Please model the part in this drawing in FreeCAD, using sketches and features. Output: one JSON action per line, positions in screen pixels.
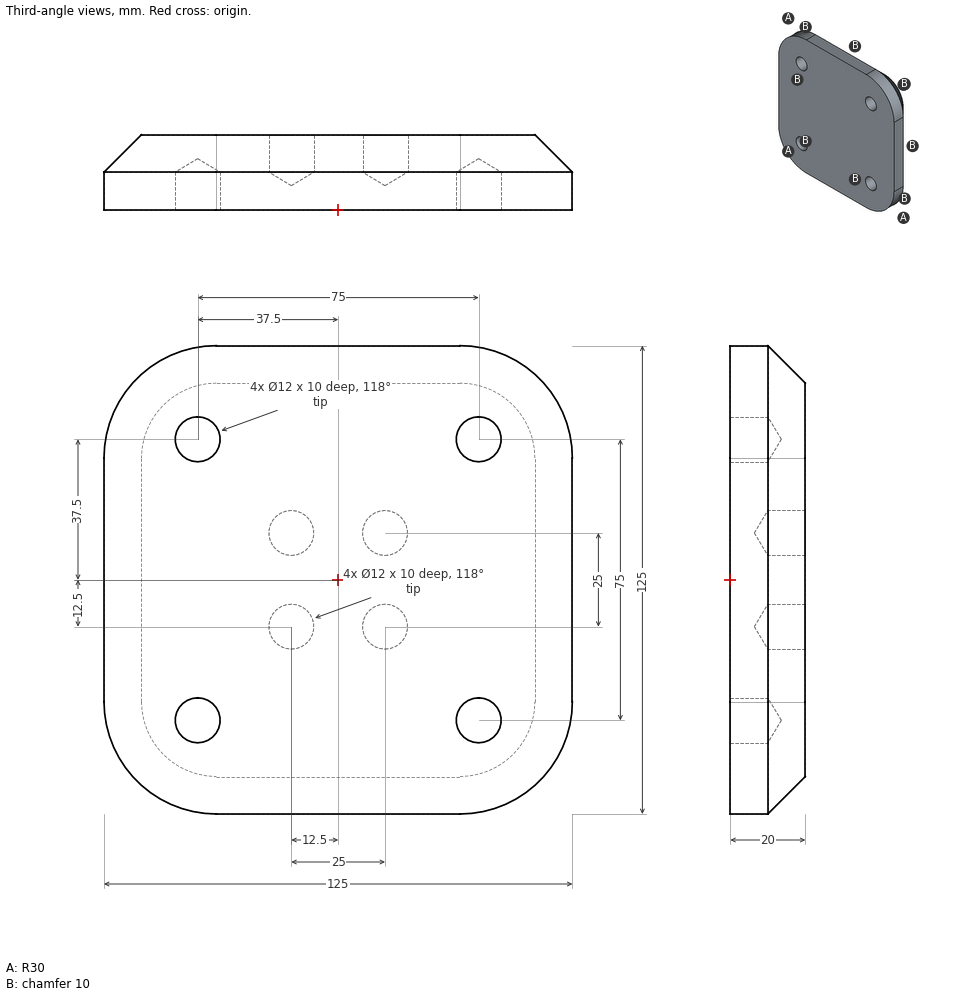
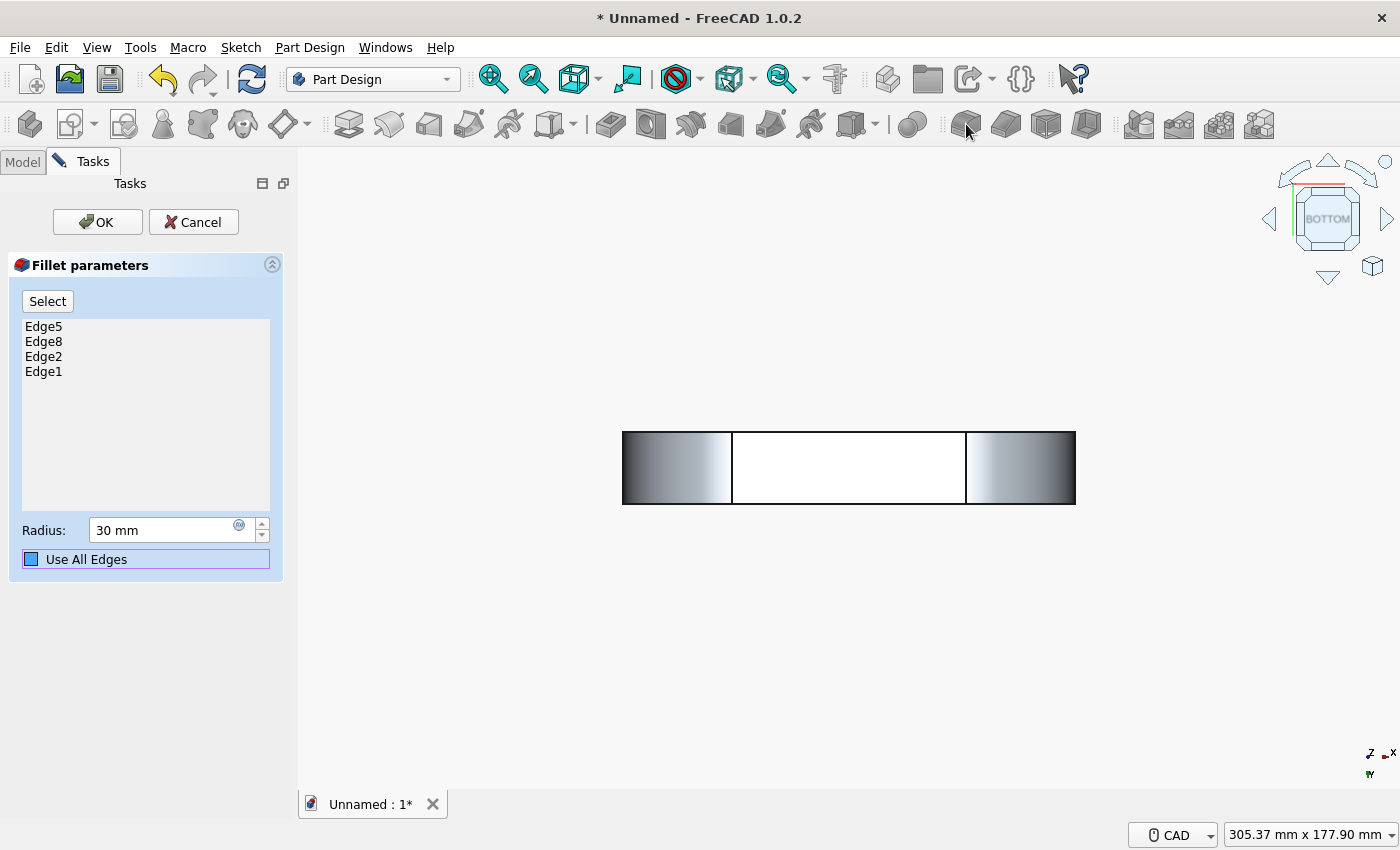
{"action": "left_click", "coordinate": [98, 222]}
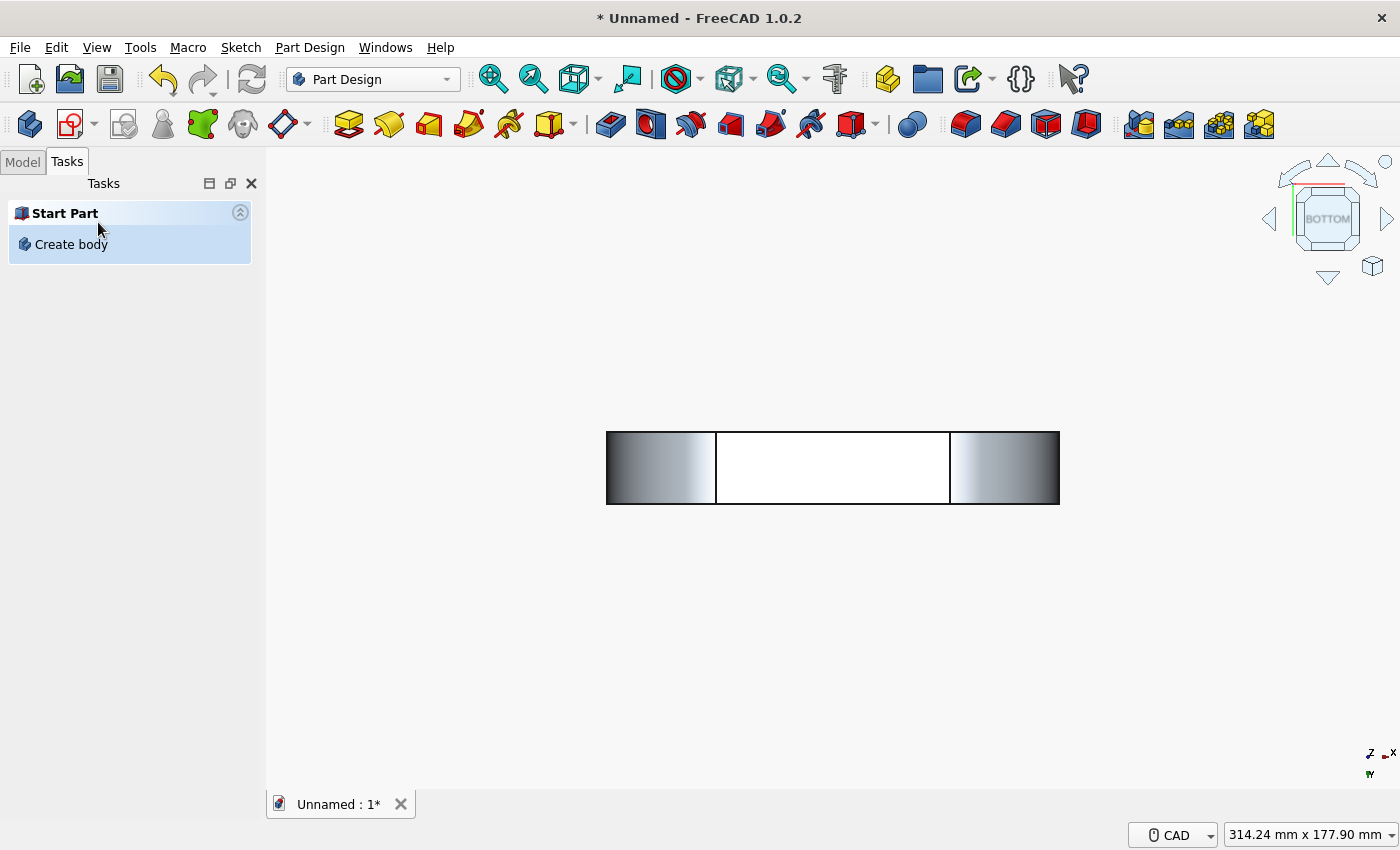
{"action": "left_click", "coordinate": [494, 80]}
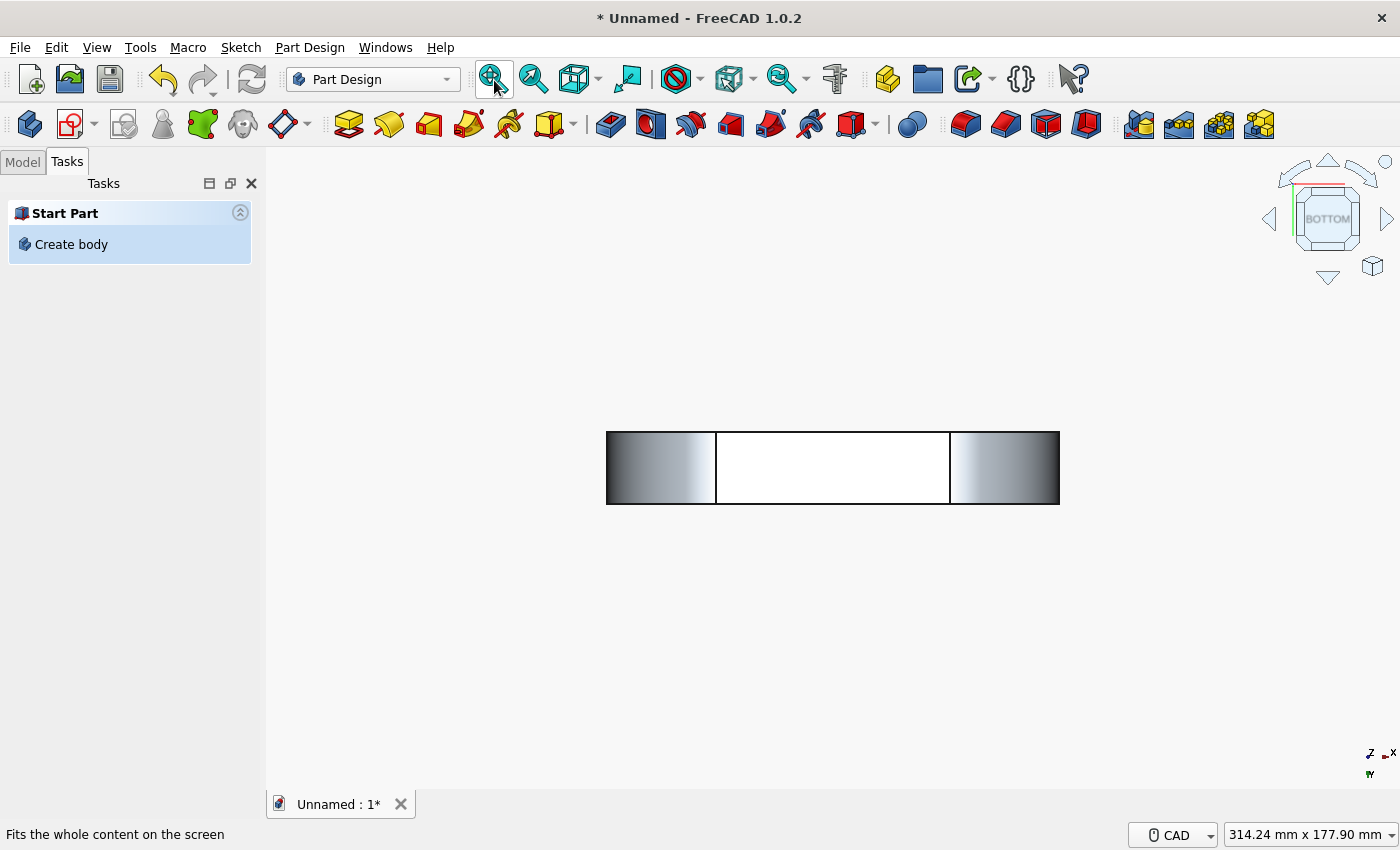
{"action": "key", "text": "0"}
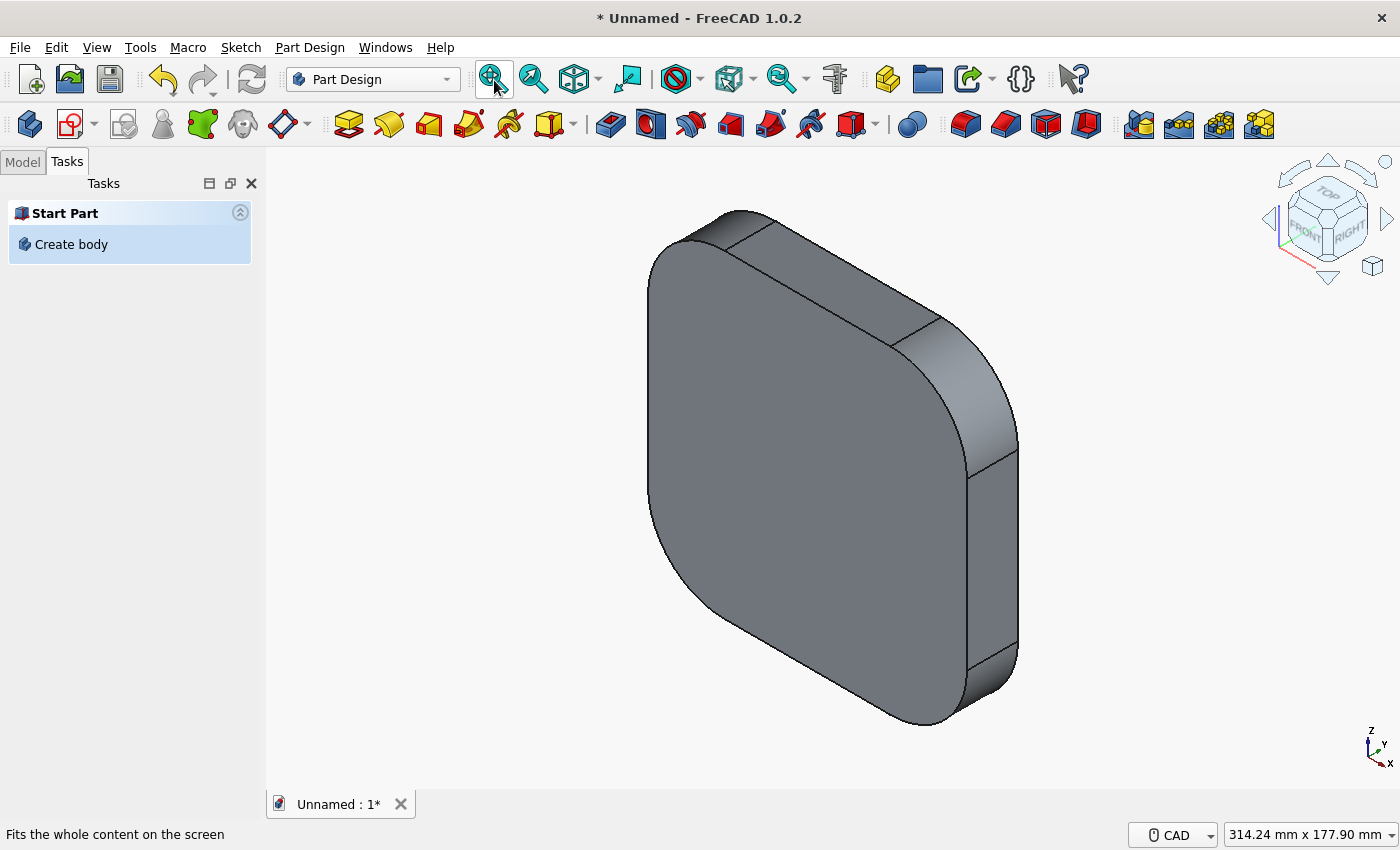
{"action": "key", "text": "2"}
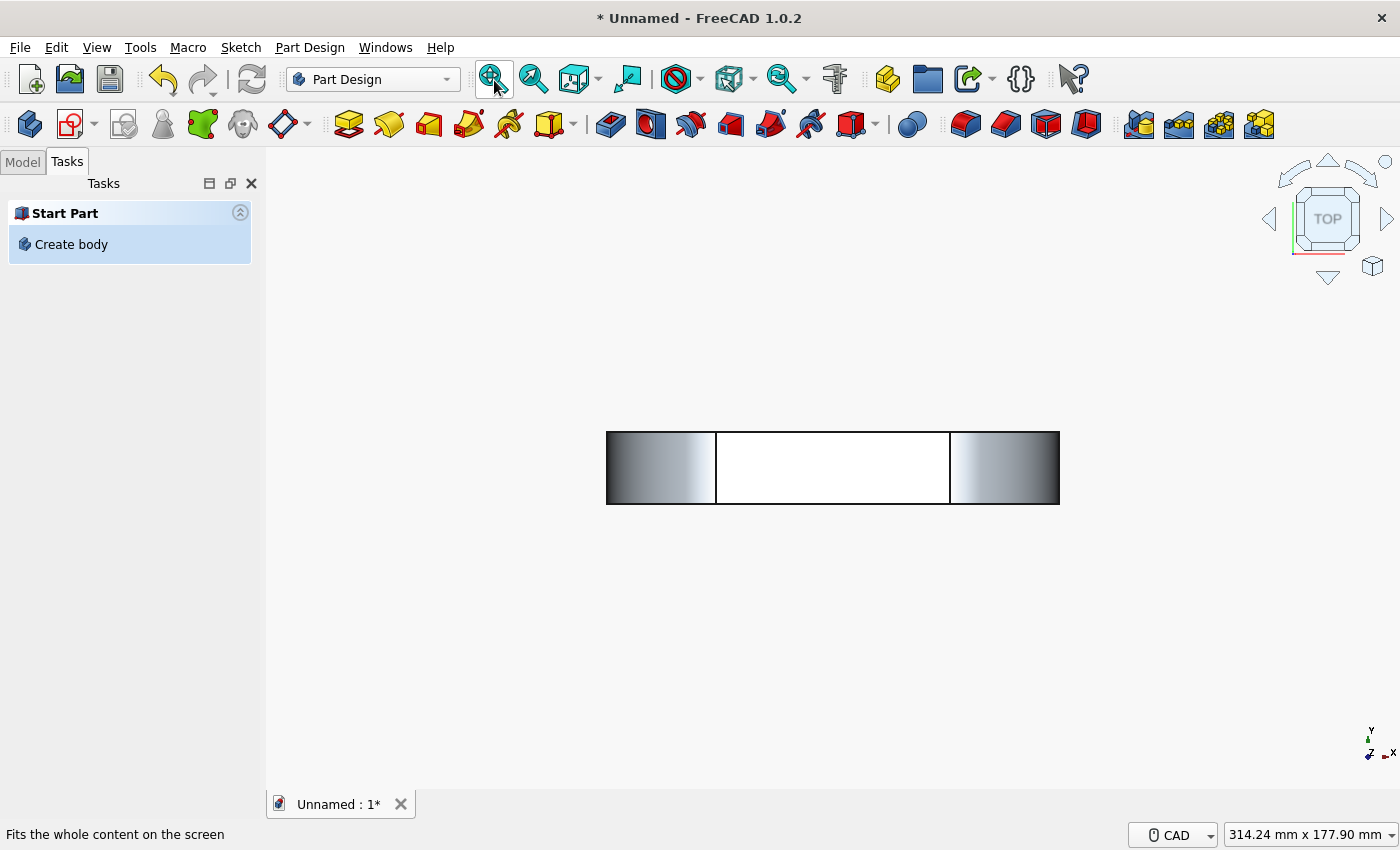
{"action": "left_click", "coordinate": [494, 80]}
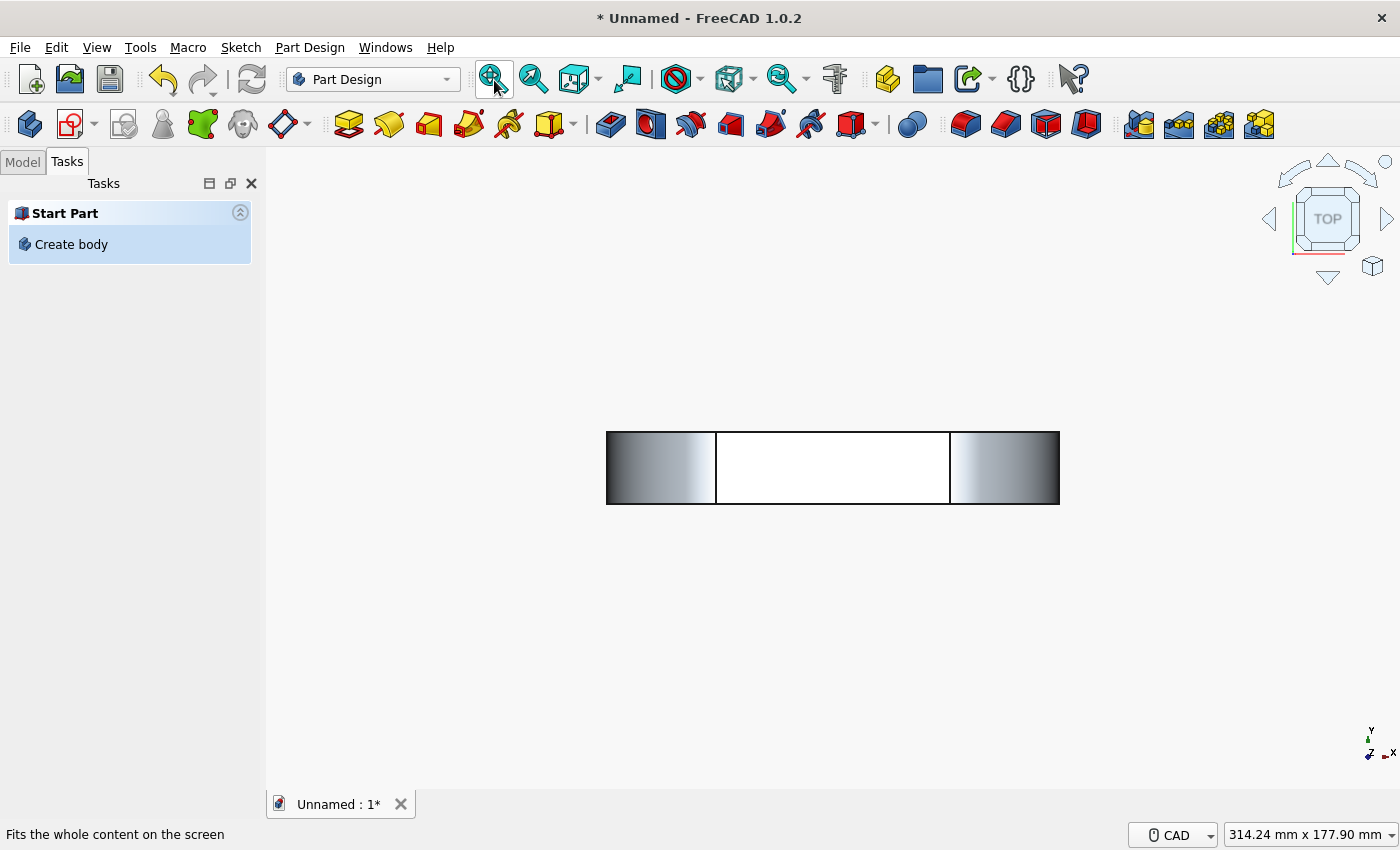
{"action": "key", "text": "1"}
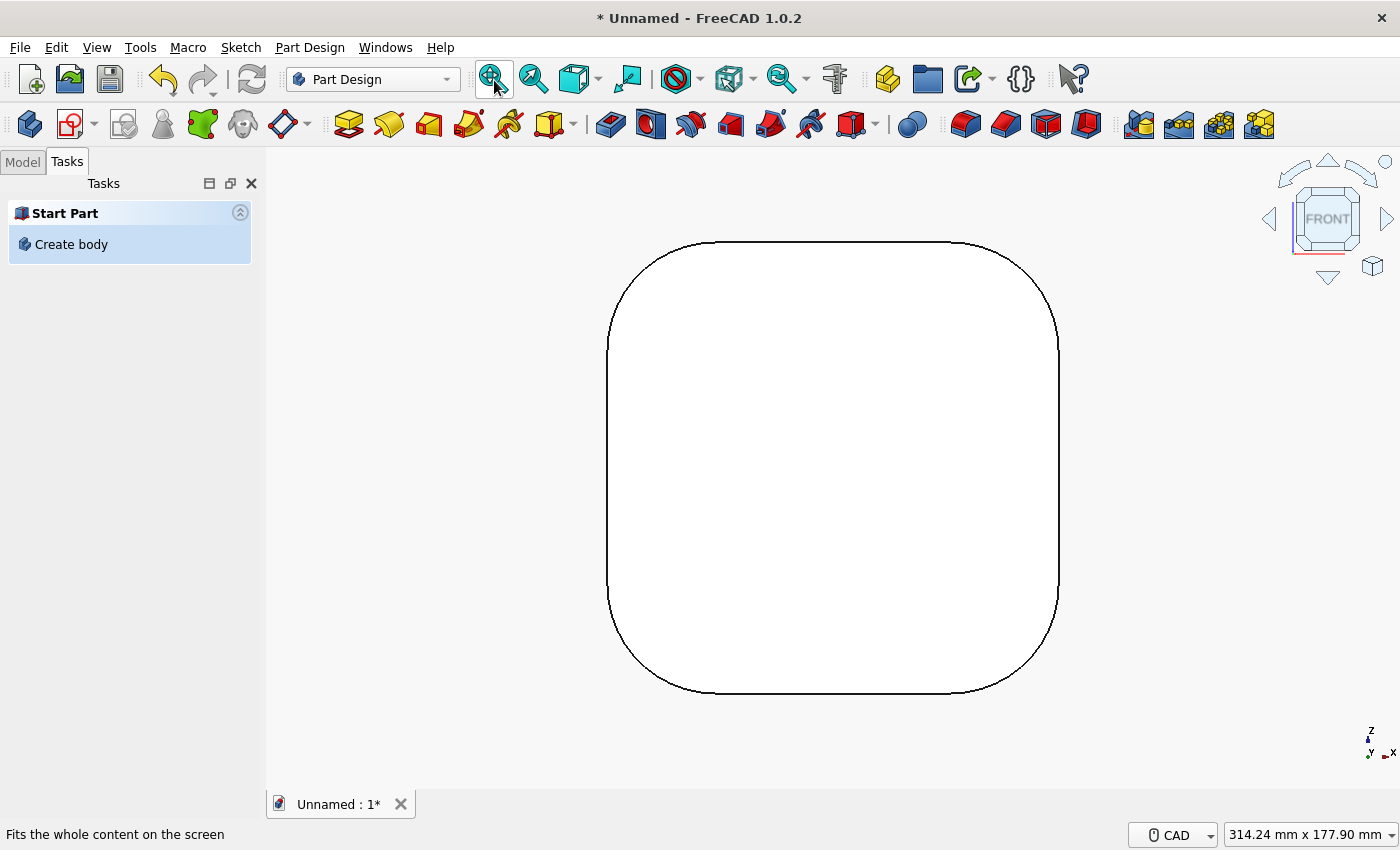
{"action": "key", "text": "3"}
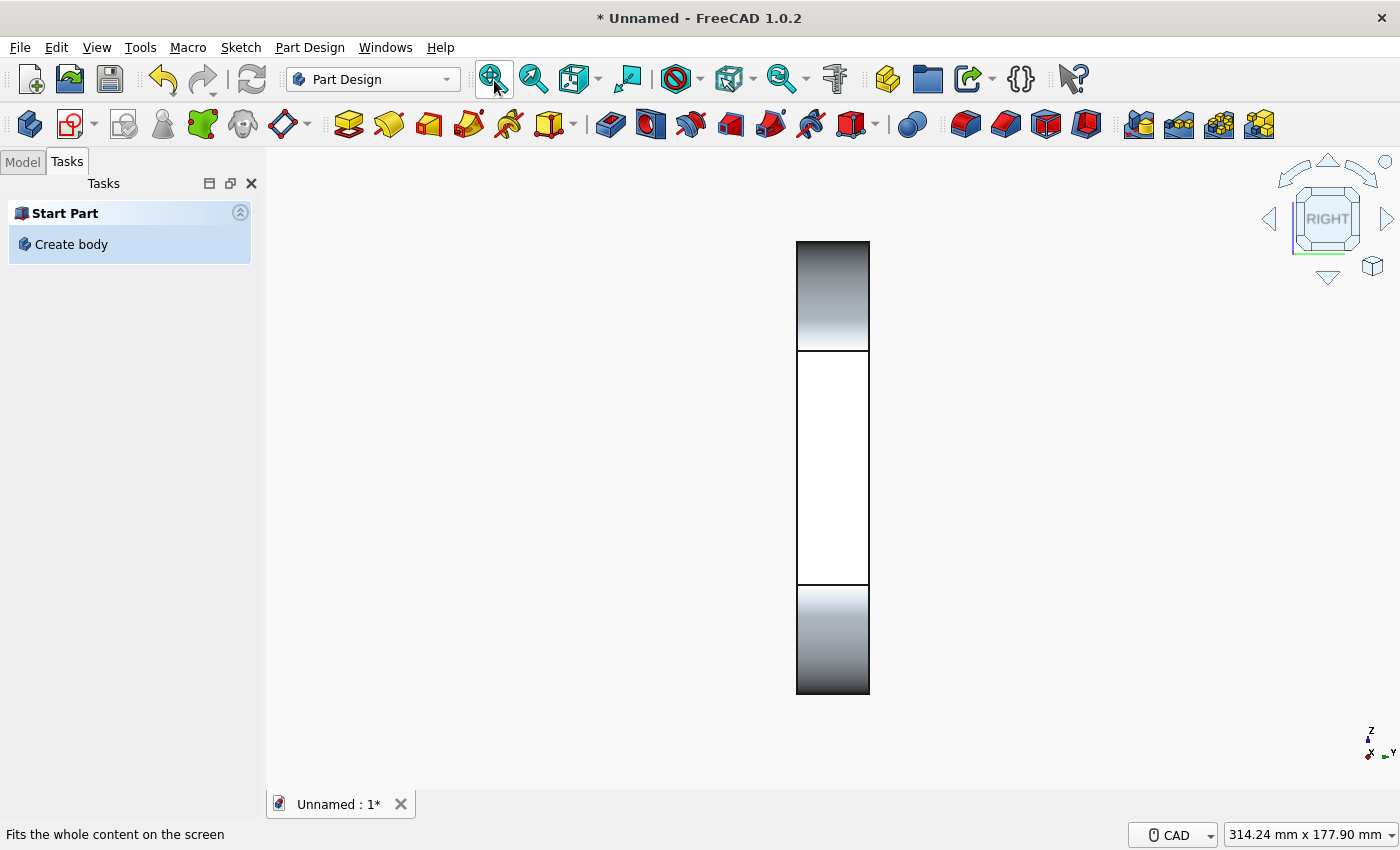
{"action": "key", "text": "5"}